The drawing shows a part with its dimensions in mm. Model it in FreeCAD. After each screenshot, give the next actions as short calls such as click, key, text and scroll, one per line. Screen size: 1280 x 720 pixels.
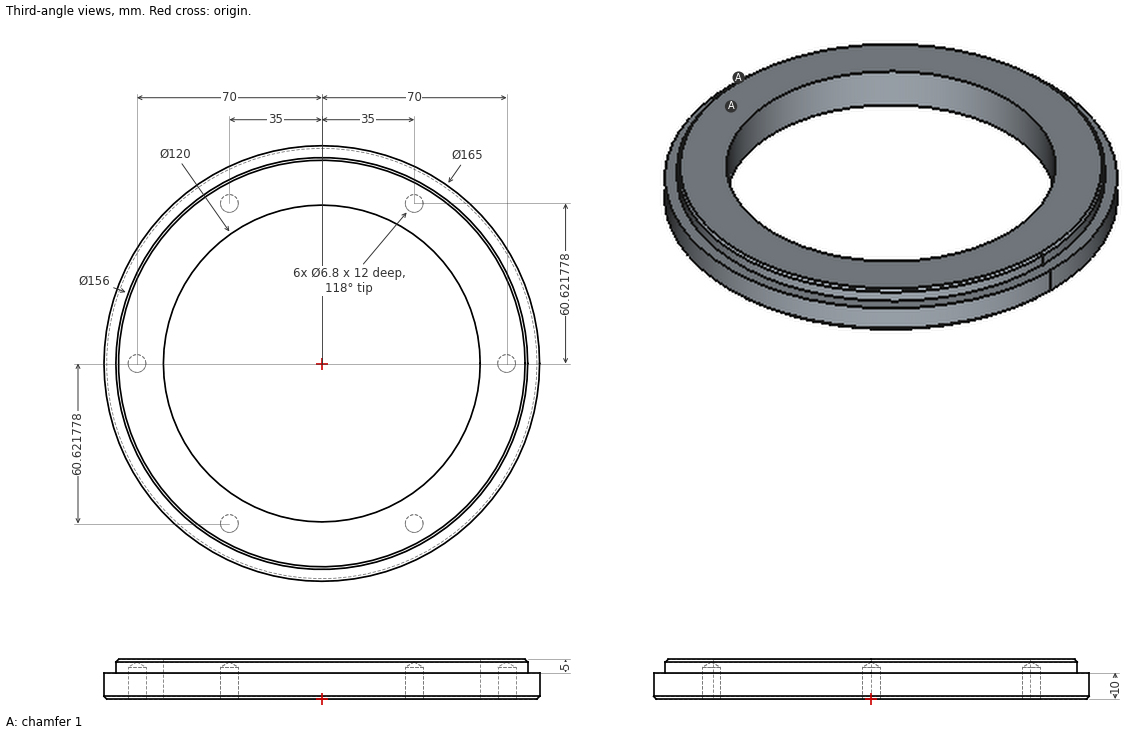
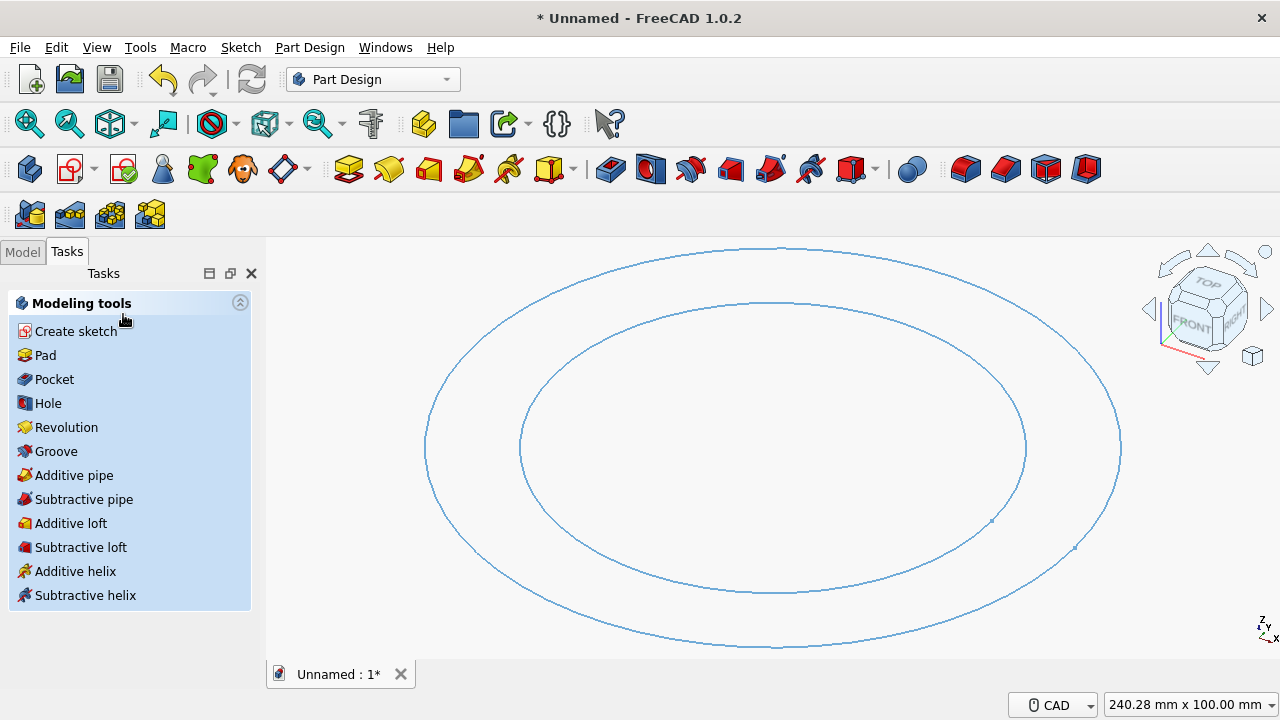
click(350, 170)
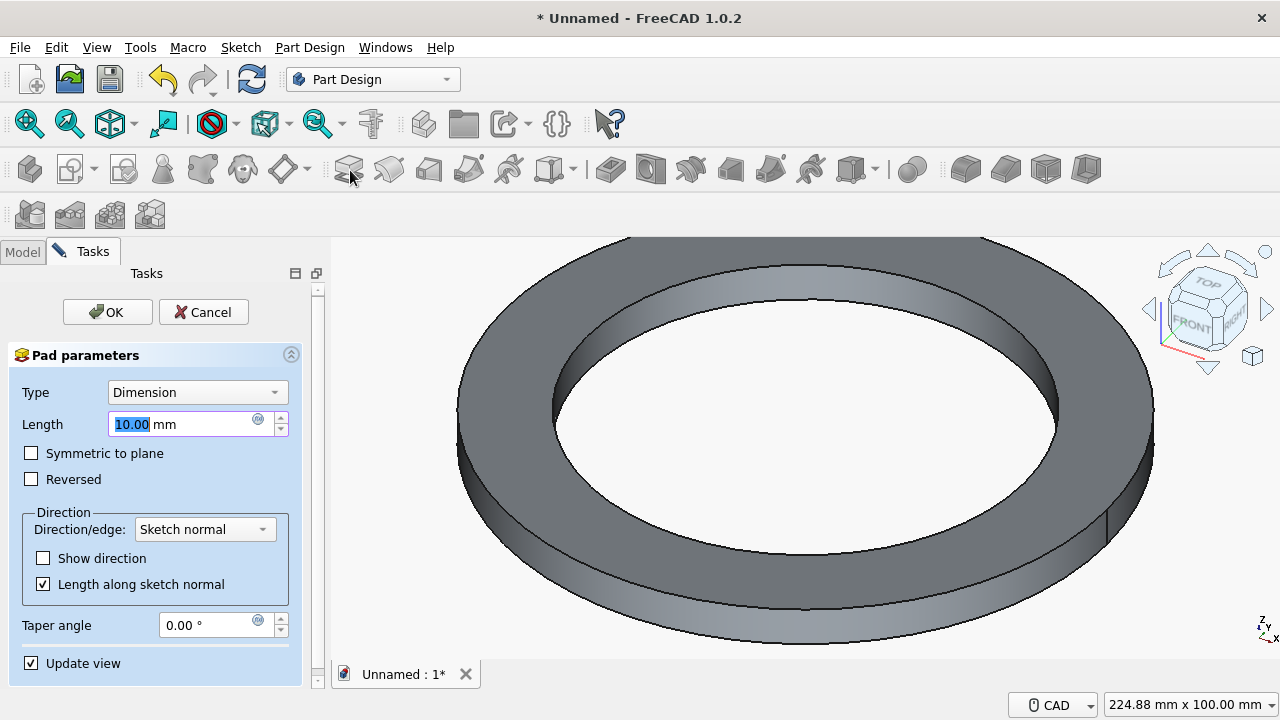
text(10)
key(Tab)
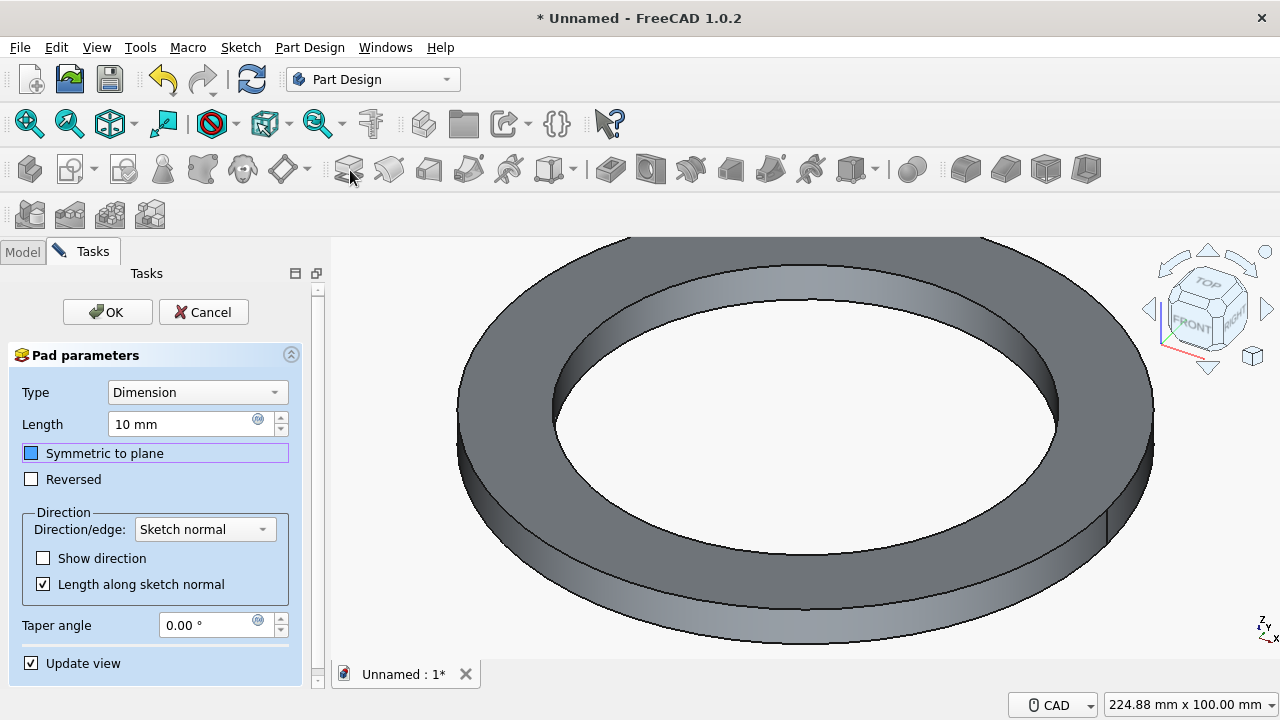
click(108, 312)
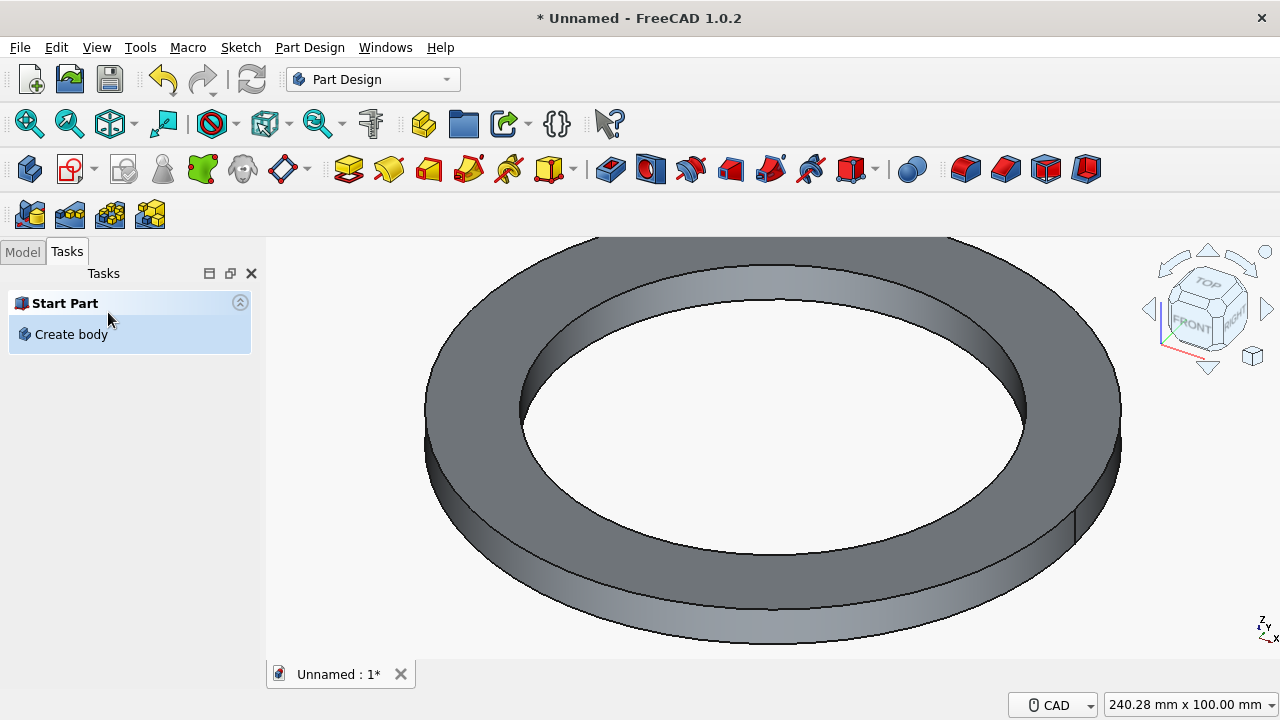
click(30, 124)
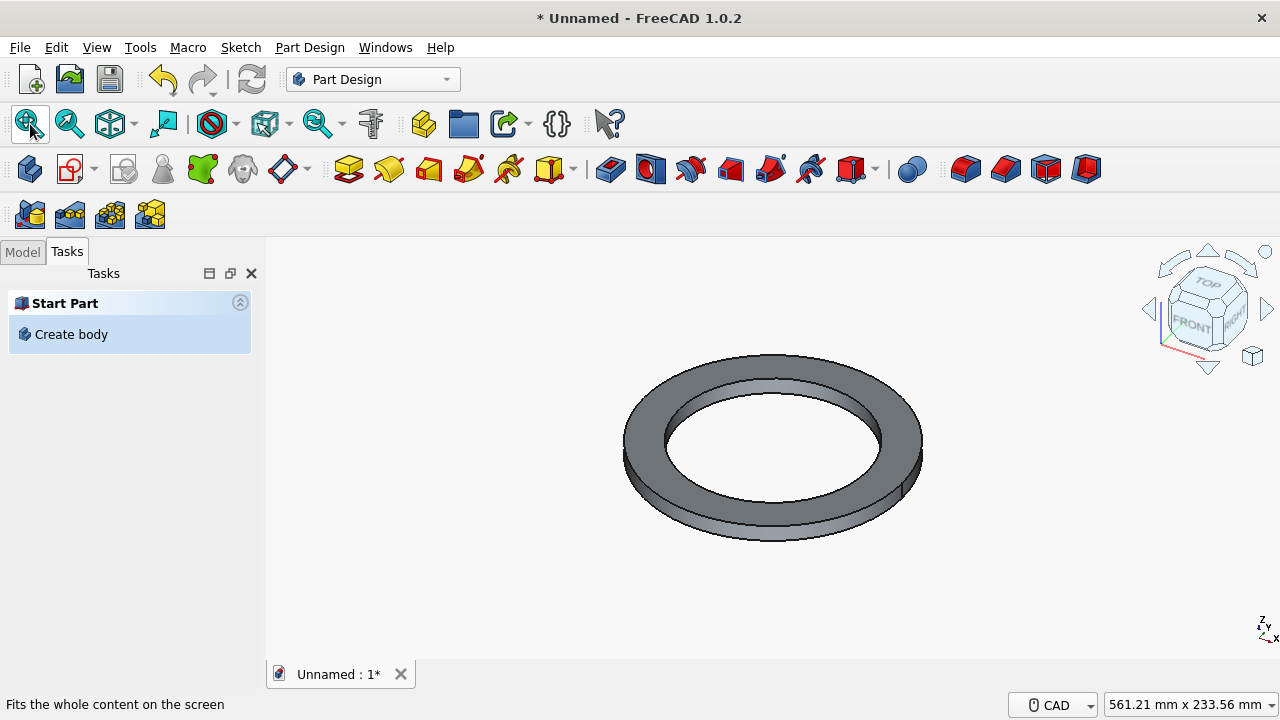
click(884, 476)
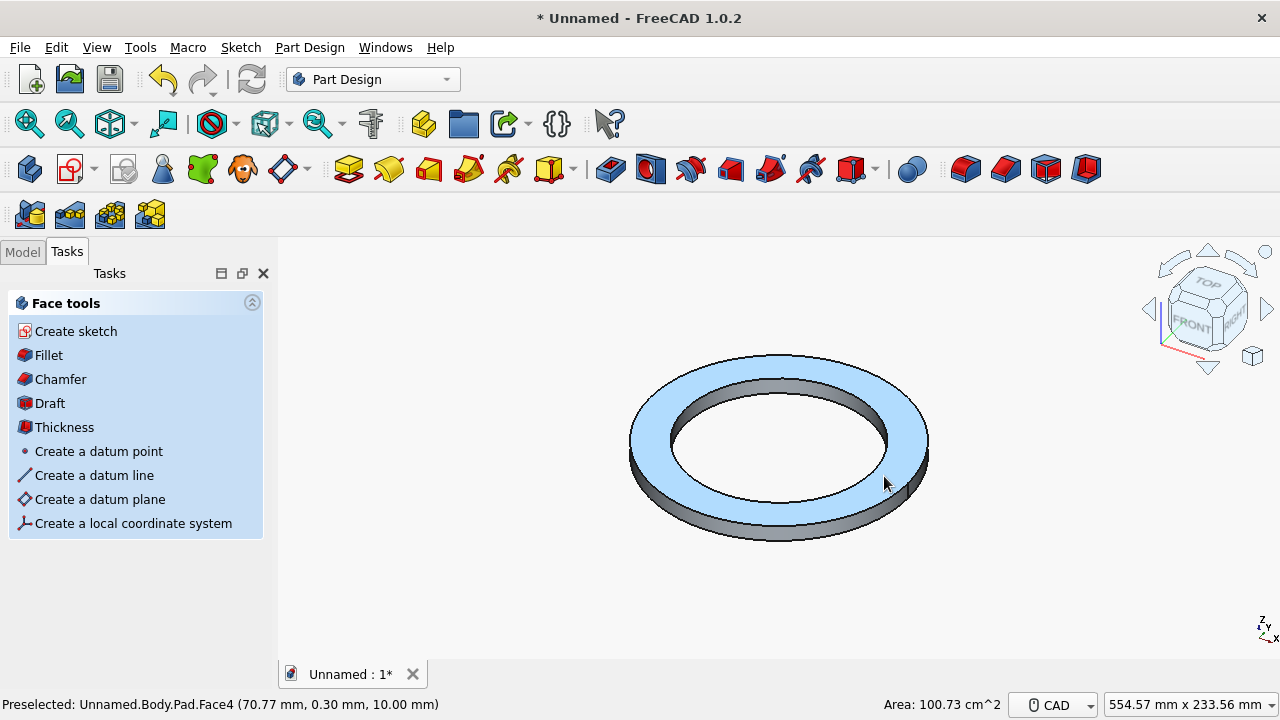
click(70, 170)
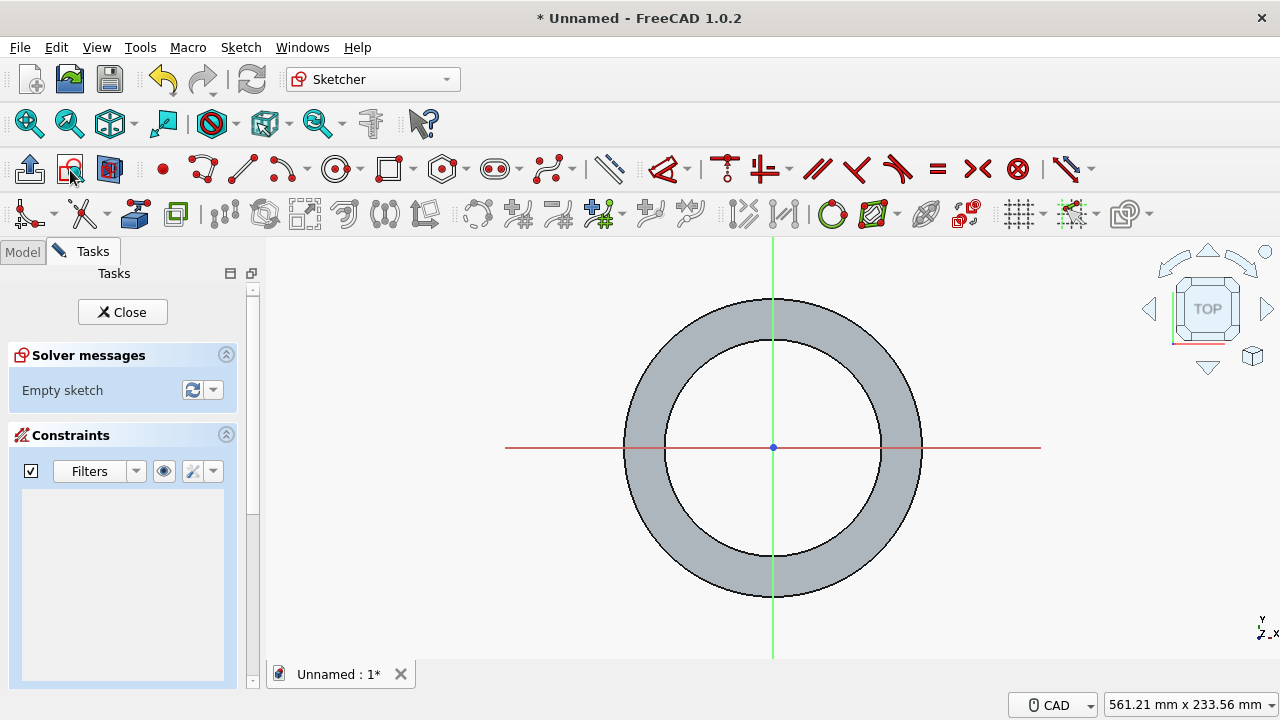
click(336, 170)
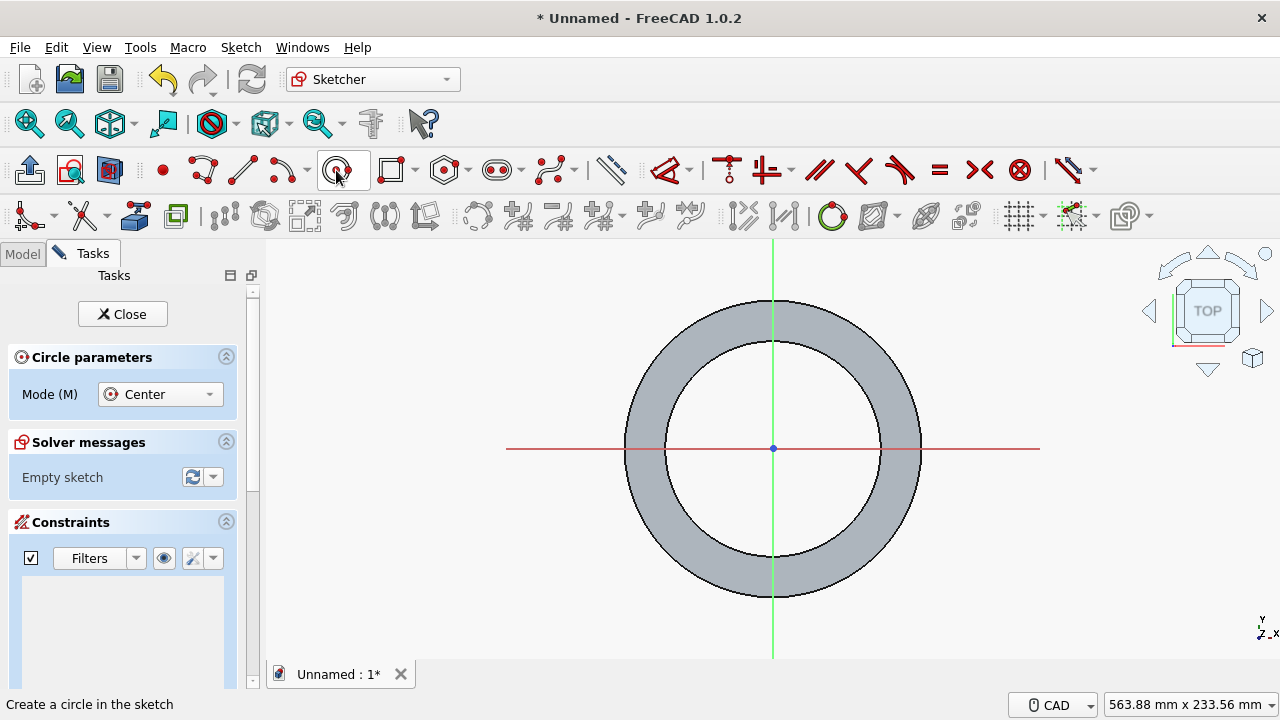
click(773, 449)
move(872, 350)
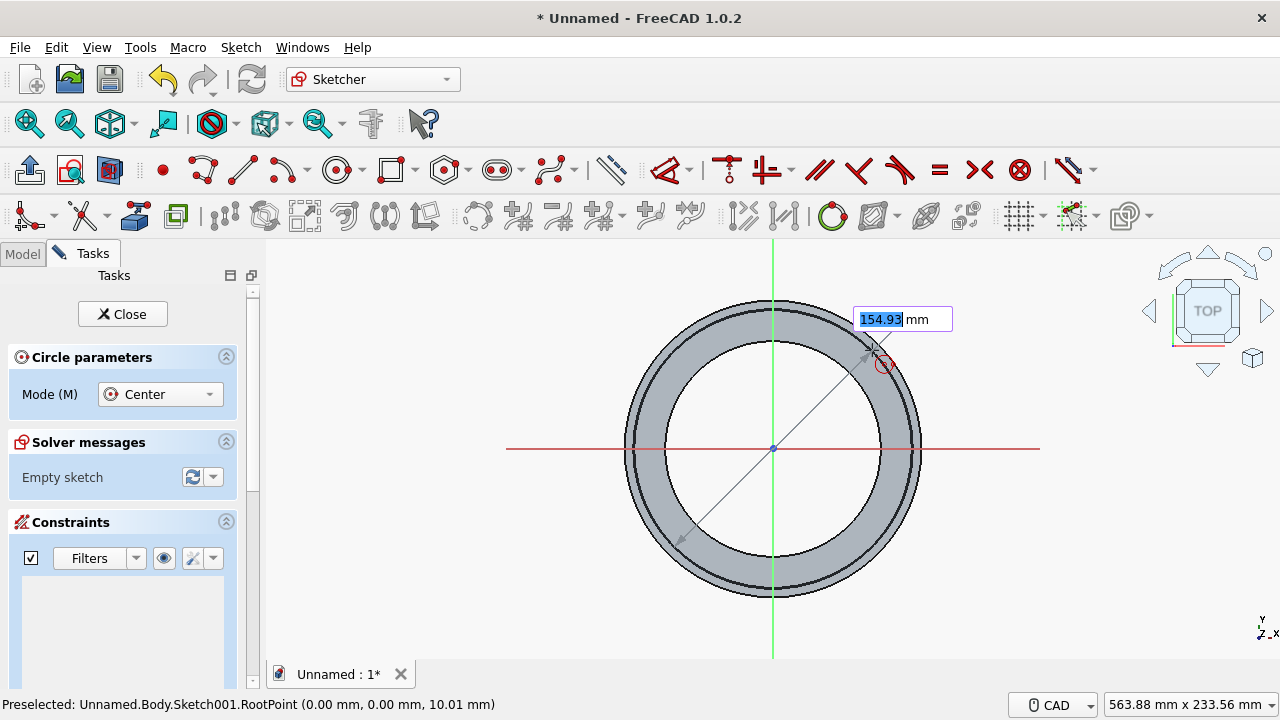
text(156)
key(Return)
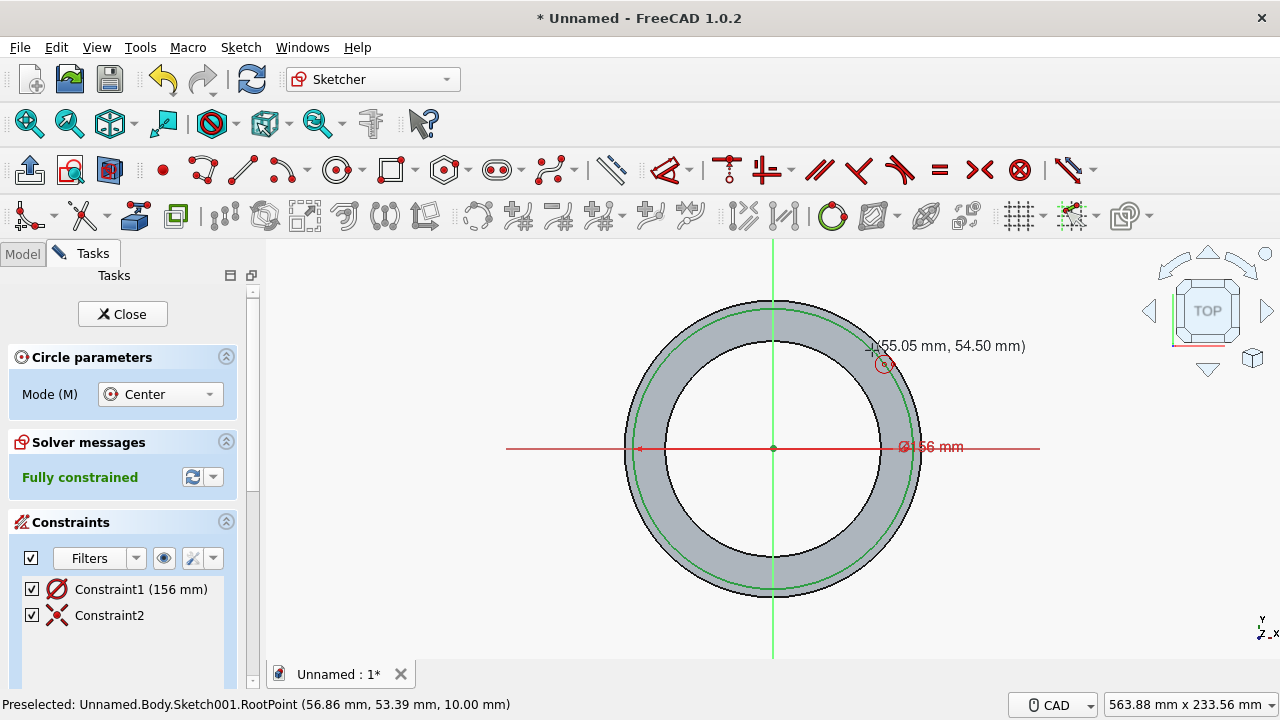
click(773, 449)
move(849, 373)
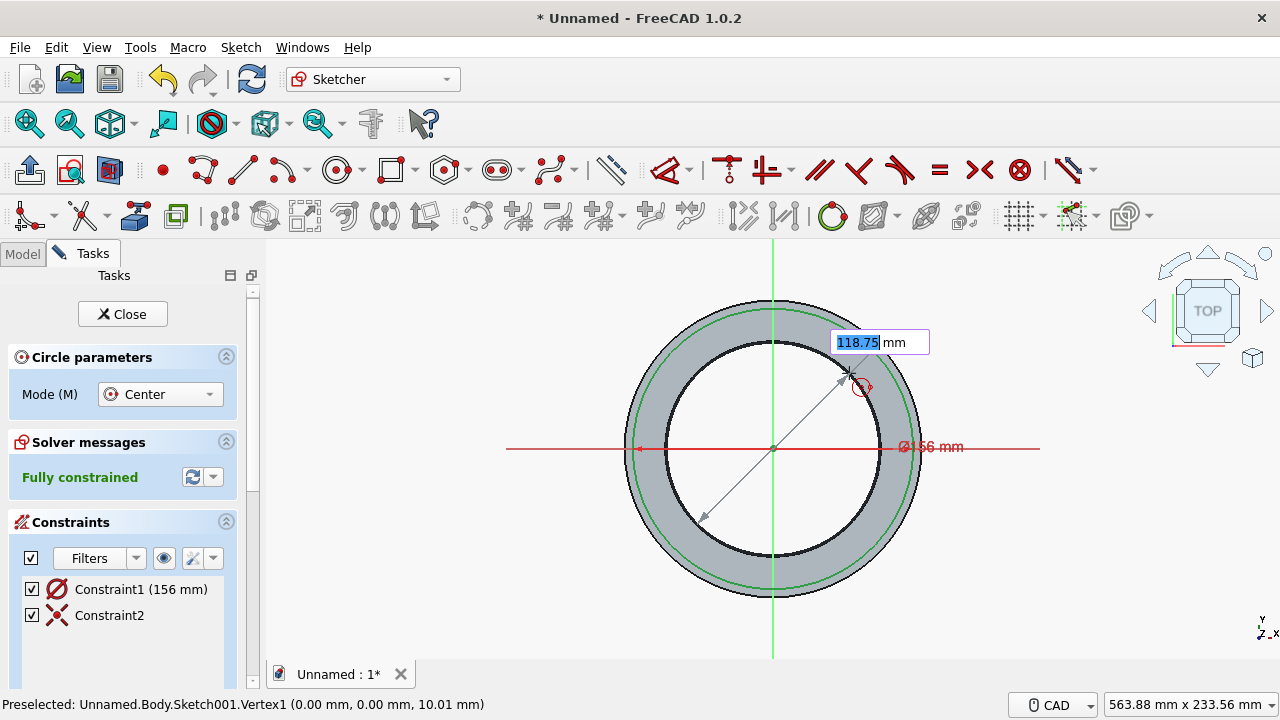
text(120)
key(Return)
key(Escape)